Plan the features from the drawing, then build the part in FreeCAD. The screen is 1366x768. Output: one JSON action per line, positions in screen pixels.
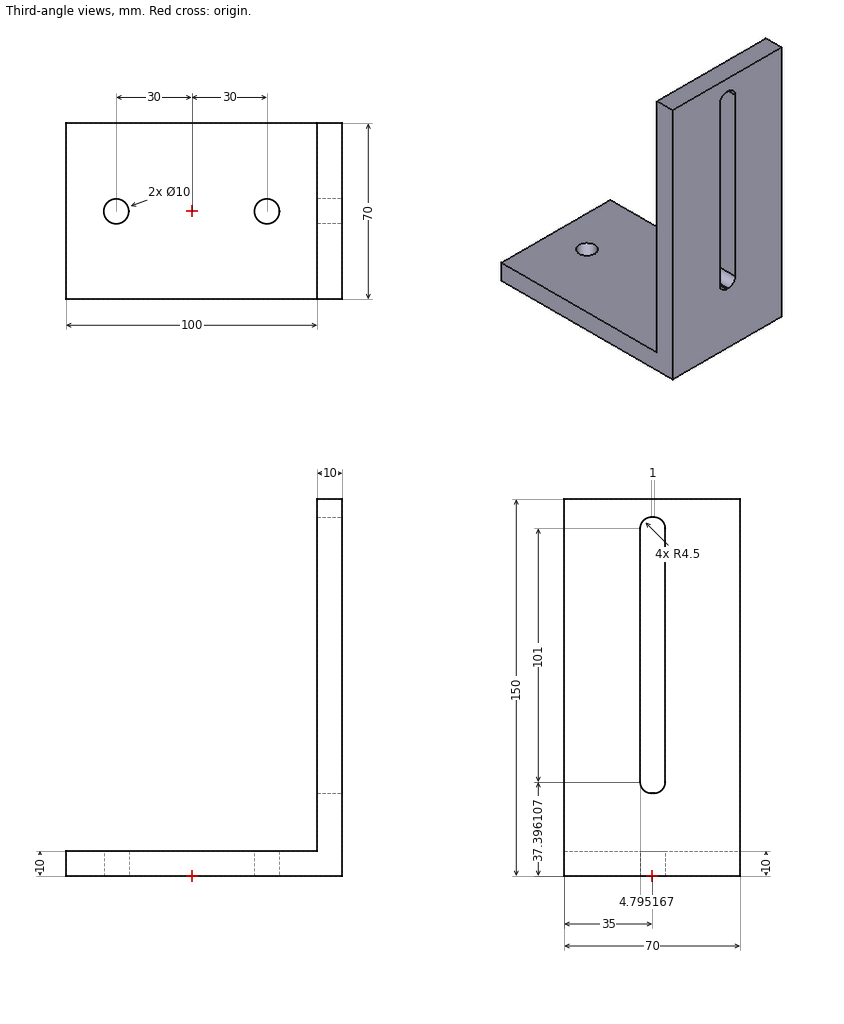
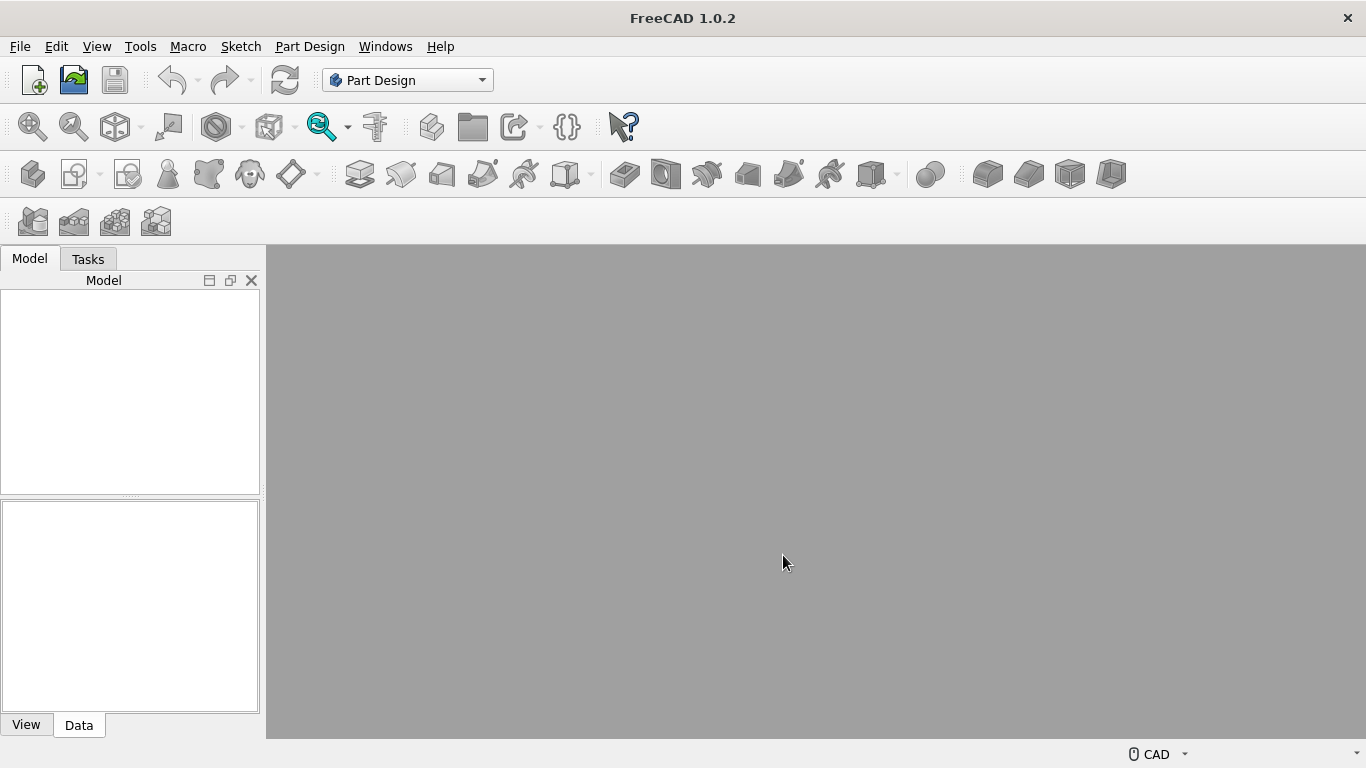
{"action": "left_click", "coordinate": [33, 80]}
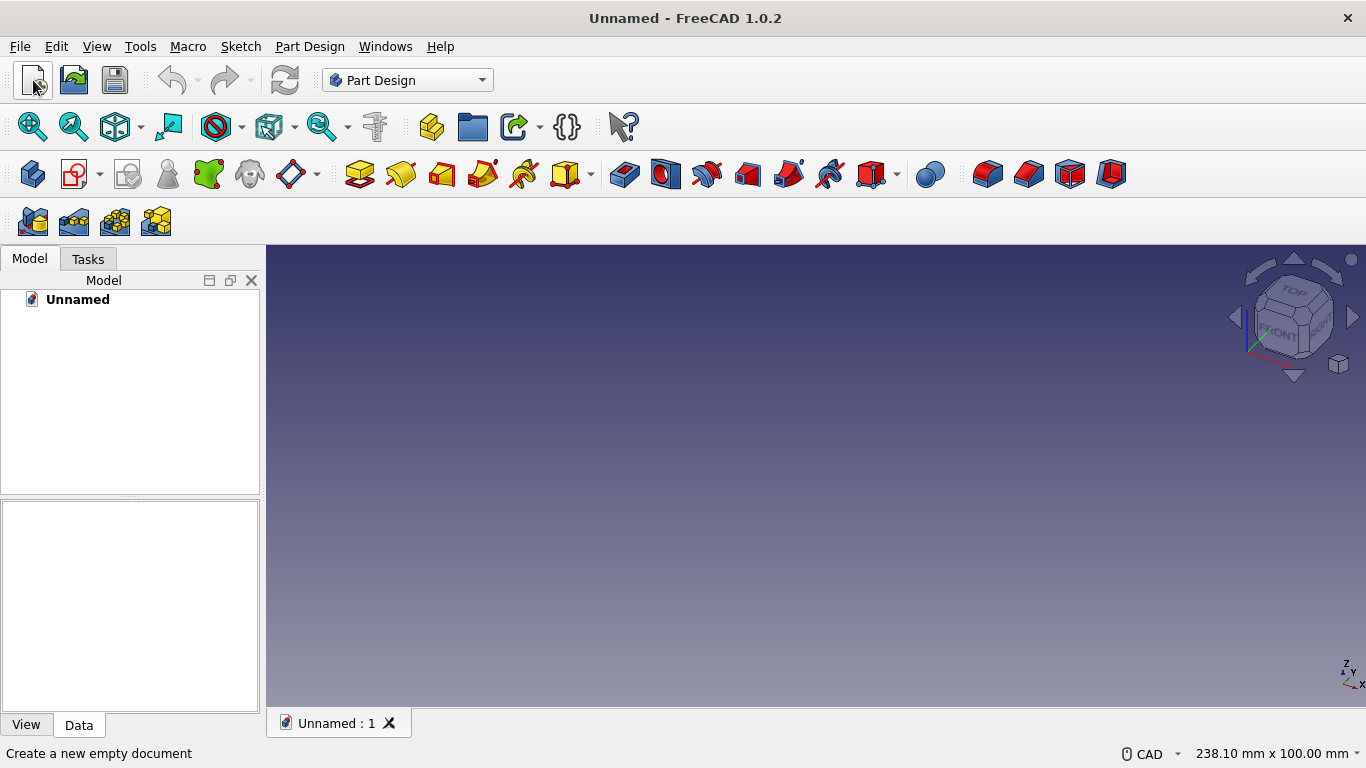
{"action": "left_click", "coordinate": [74, 174]}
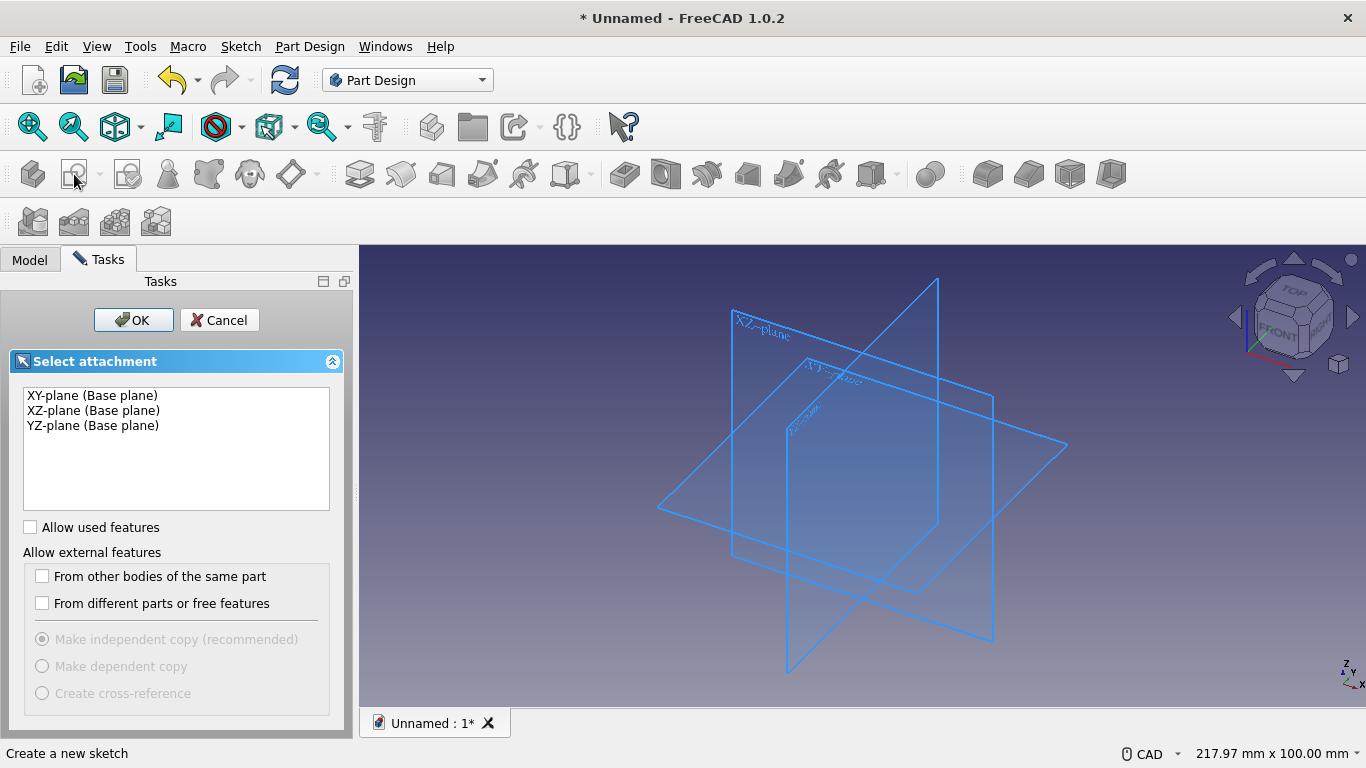
{"action": "left_click", "coordinate": [84, 396]}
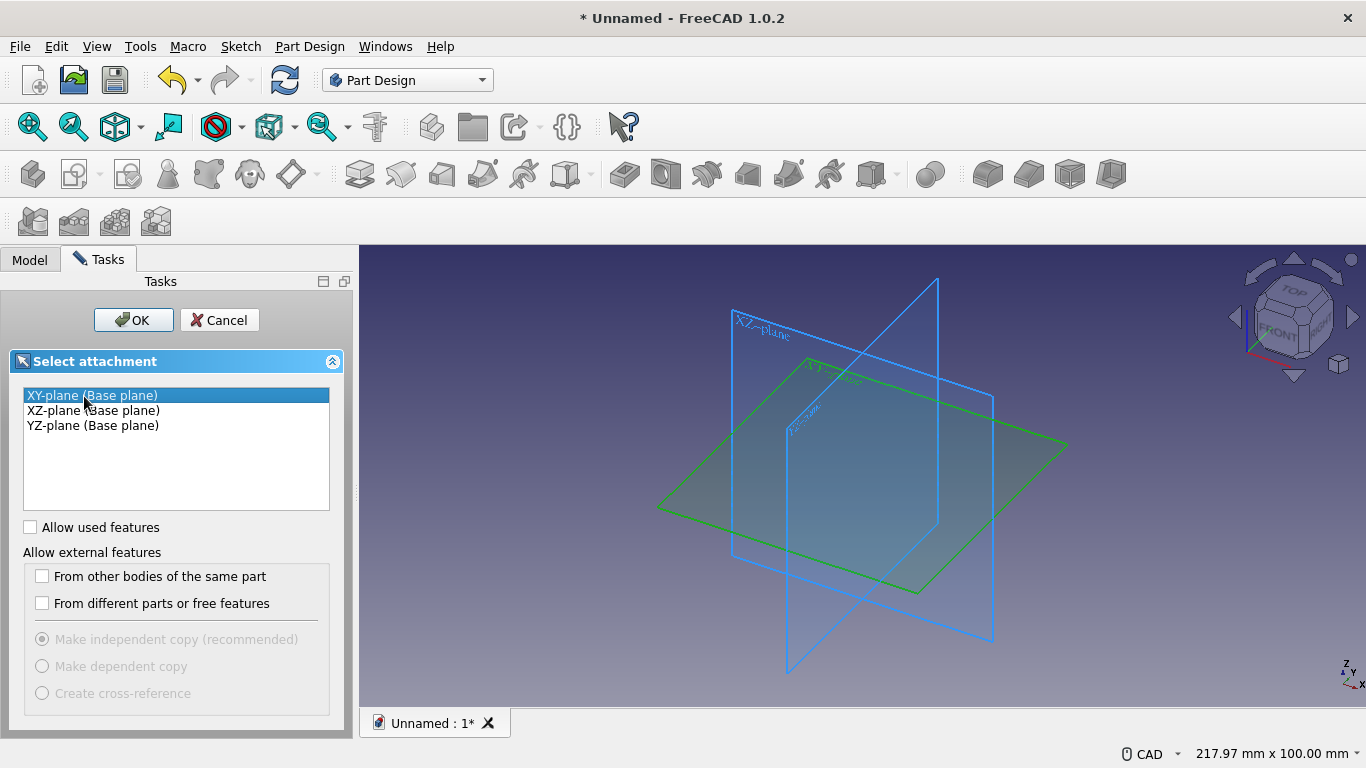
{"action": "left_click", "coordinate": [134, 320]}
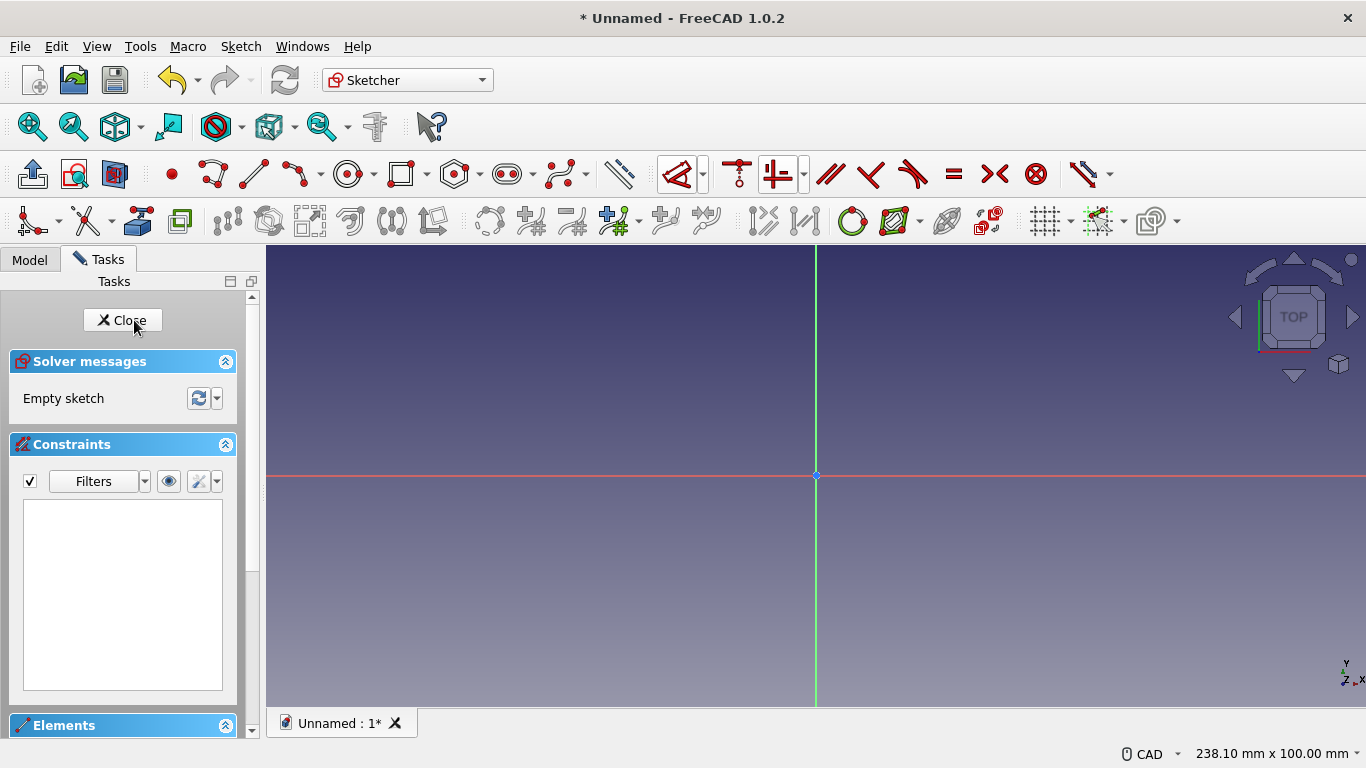
{"action": "key", "text": "g v"}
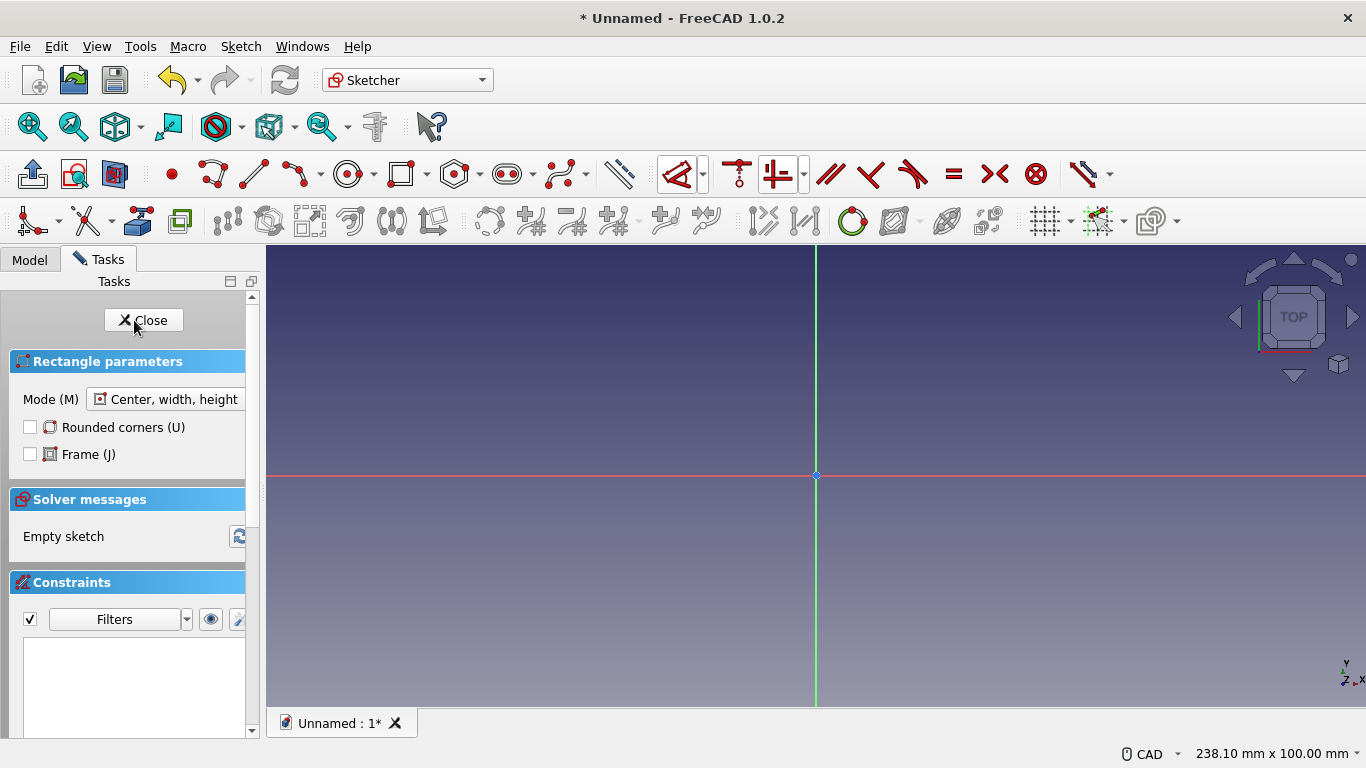
{"action": "left_click", "coordinate": [816, 476]}
{"action": "left_click", "coordinate": [1047, 314]}
{"action": "key", "text": "Escape"}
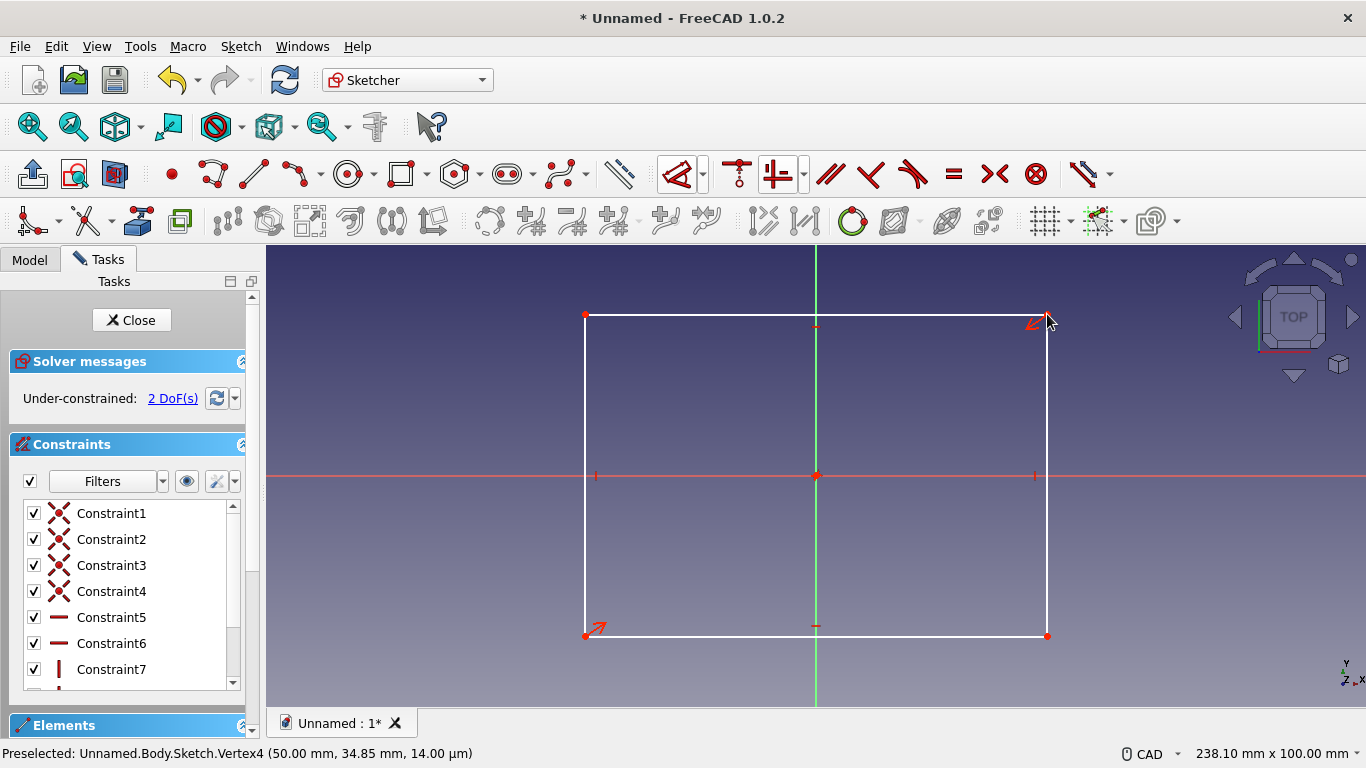
{"action": "left_click", "coordinate": [1047, 540]}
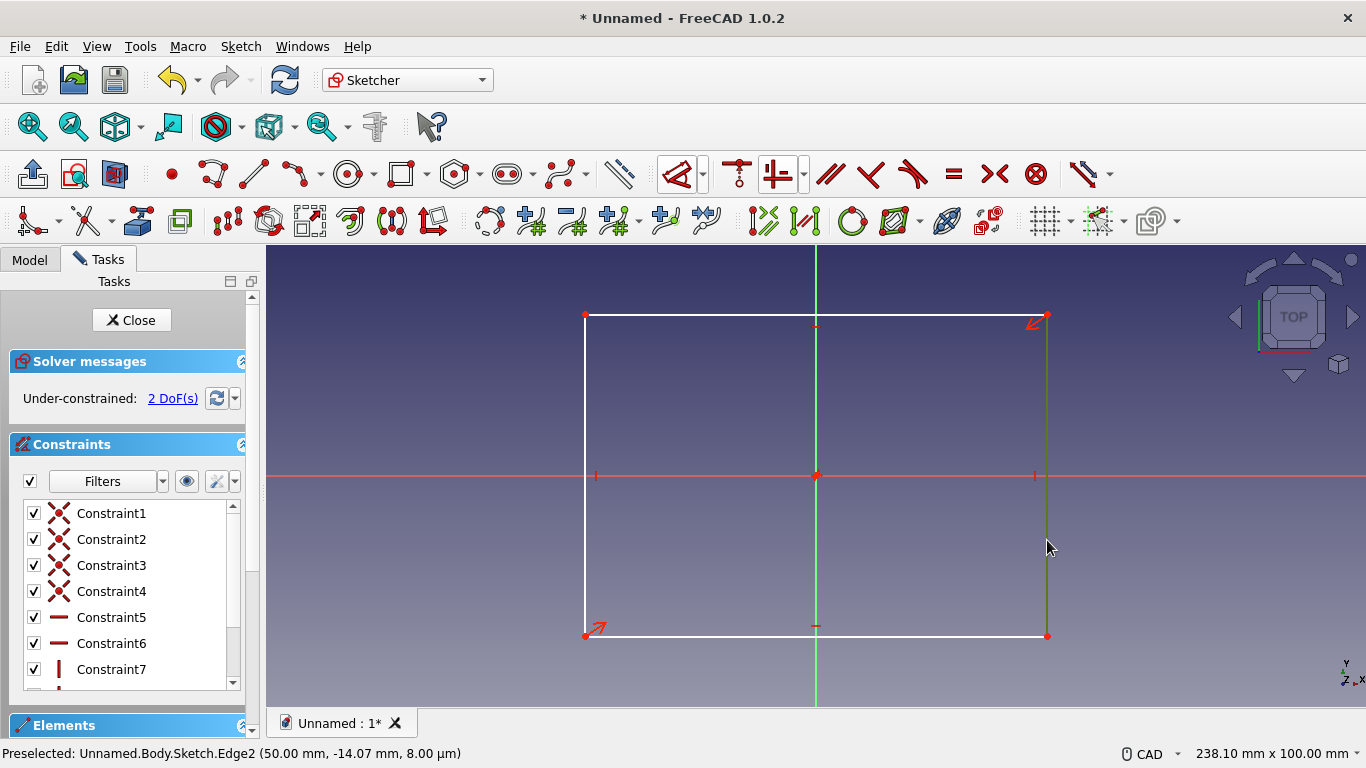
{"action": "left_click", "coordinate": [702, 174]}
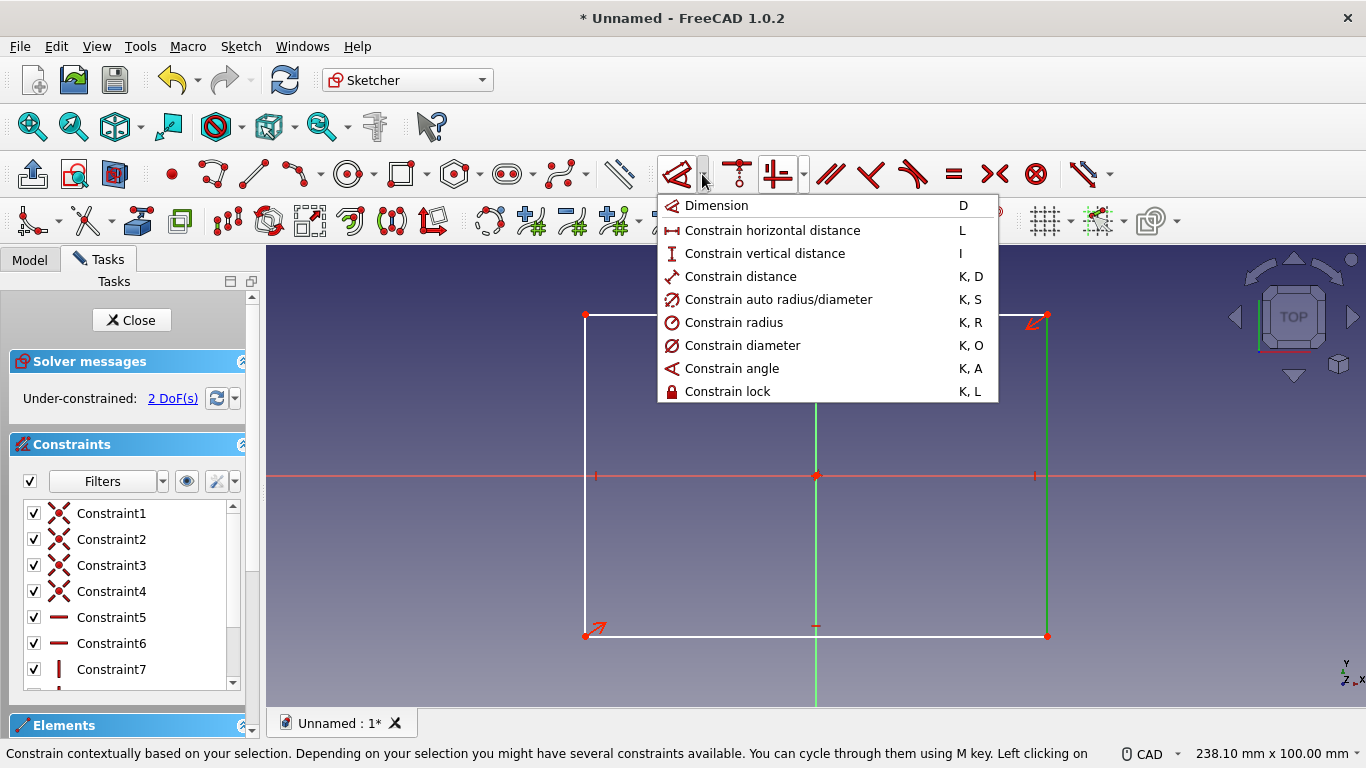
{"action": "left_click", "coordinate": [828, 254]}